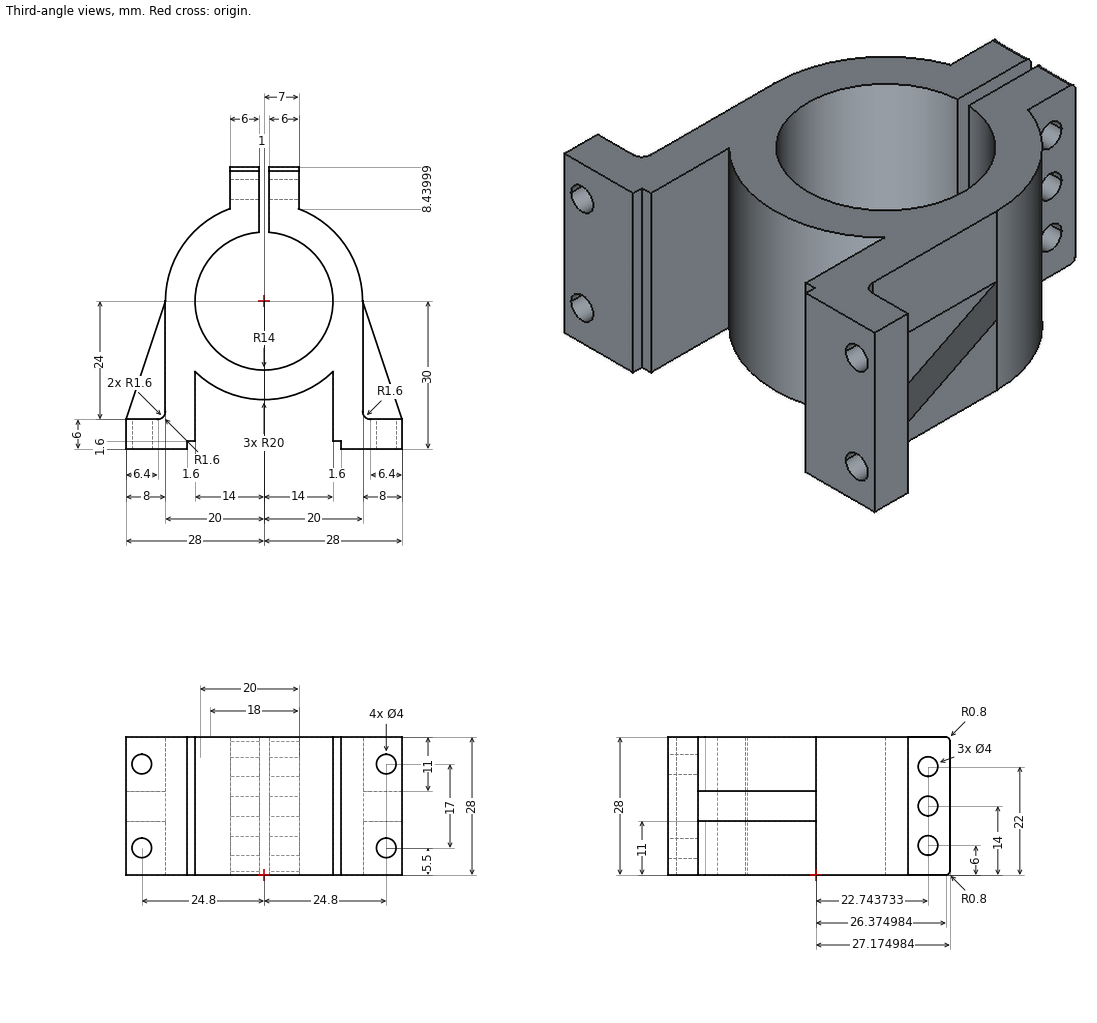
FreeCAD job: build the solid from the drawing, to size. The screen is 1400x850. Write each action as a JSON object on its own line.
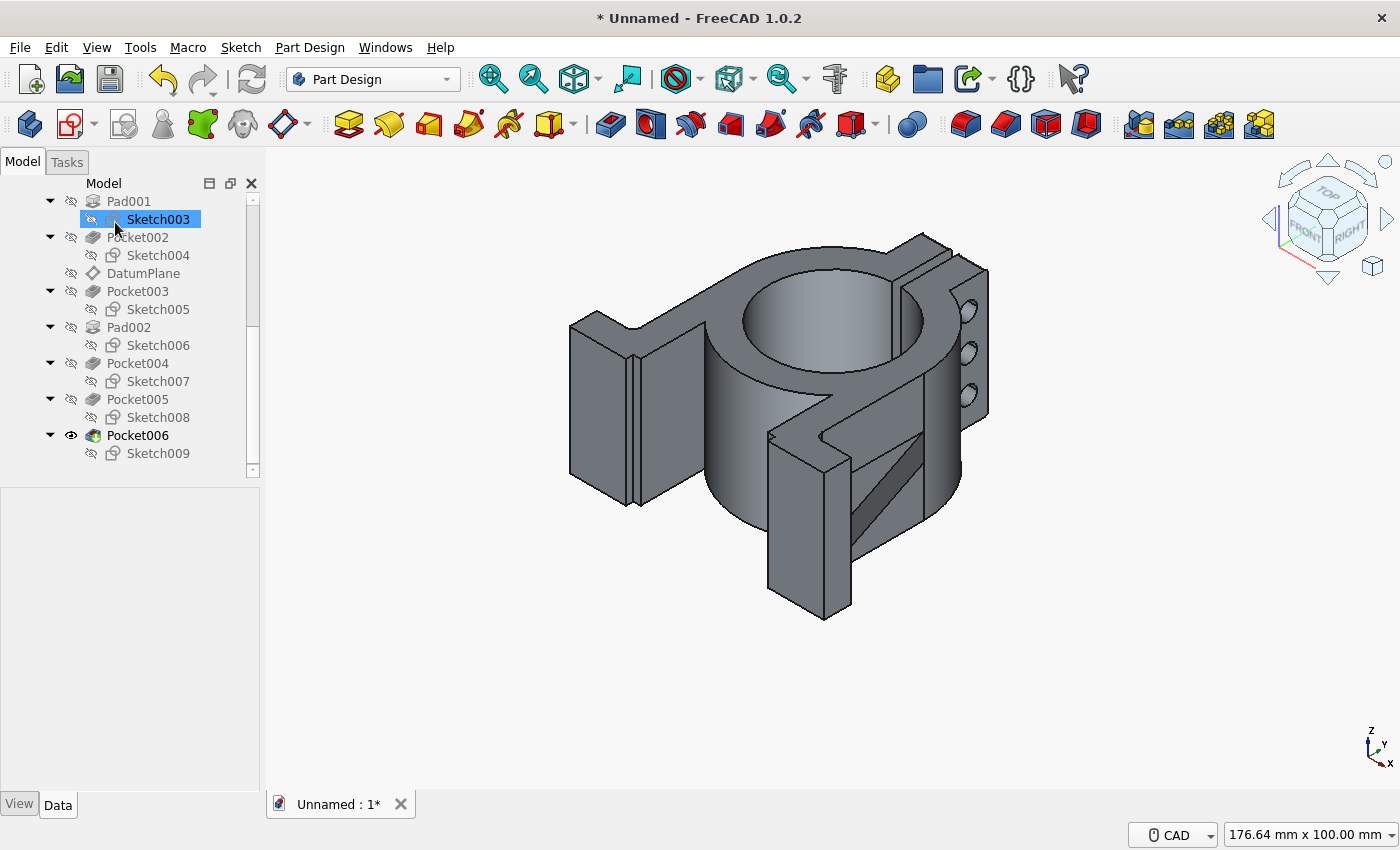
{"action": "key", "text": "4"}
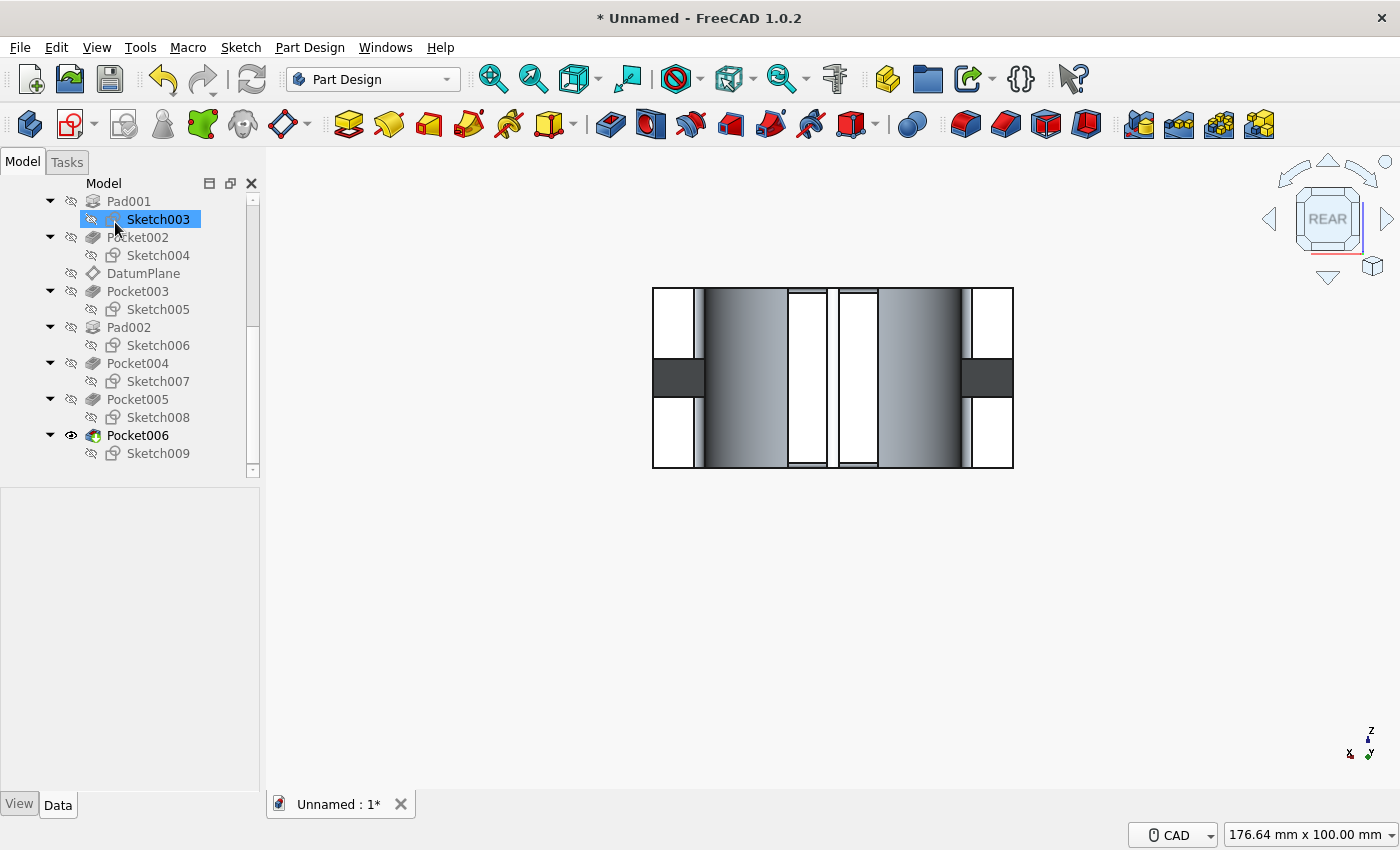
{"action": "left_click", "coordinate": [494, 80]}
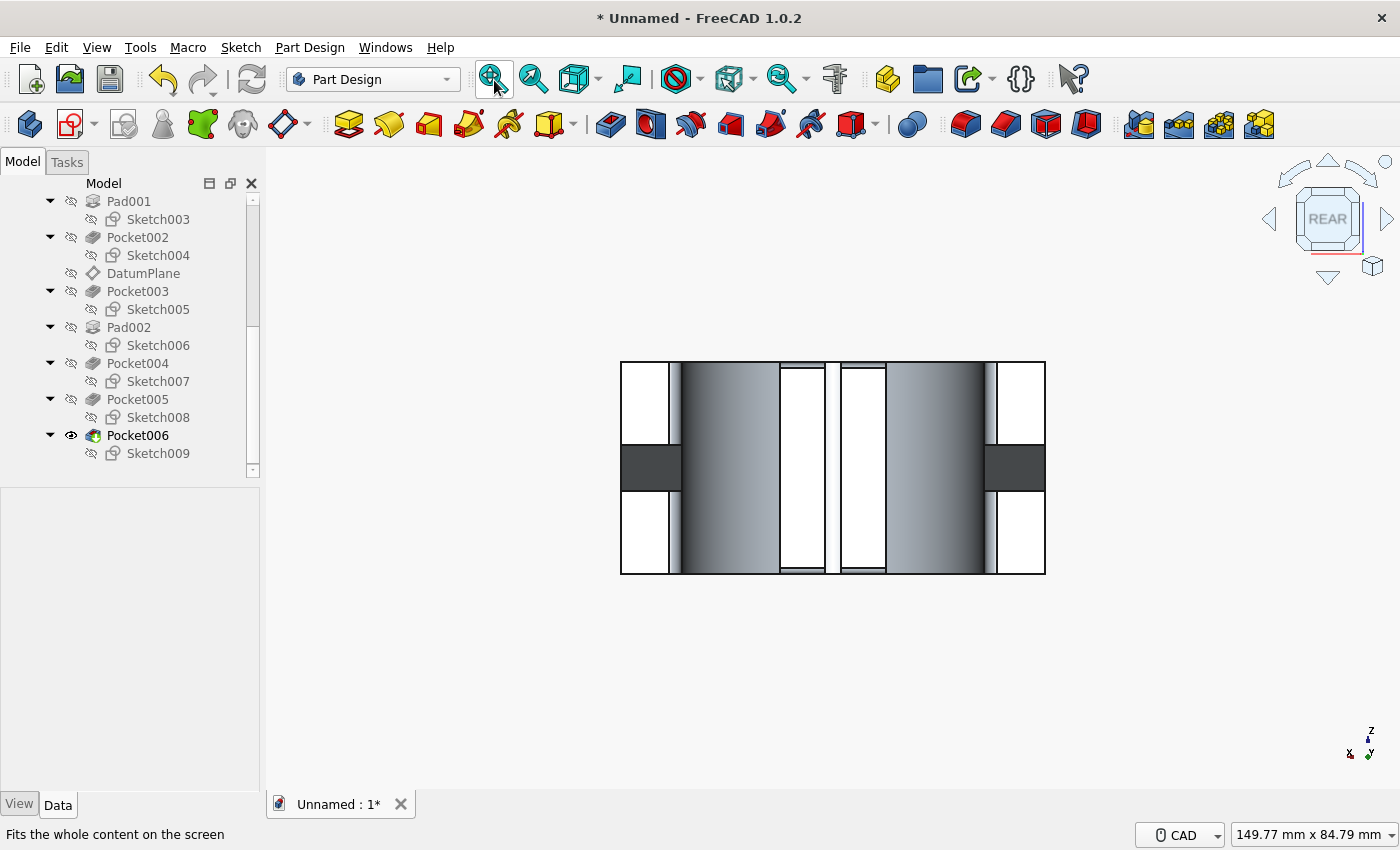
{"action": "left_click", "coordinate": [645, 519]}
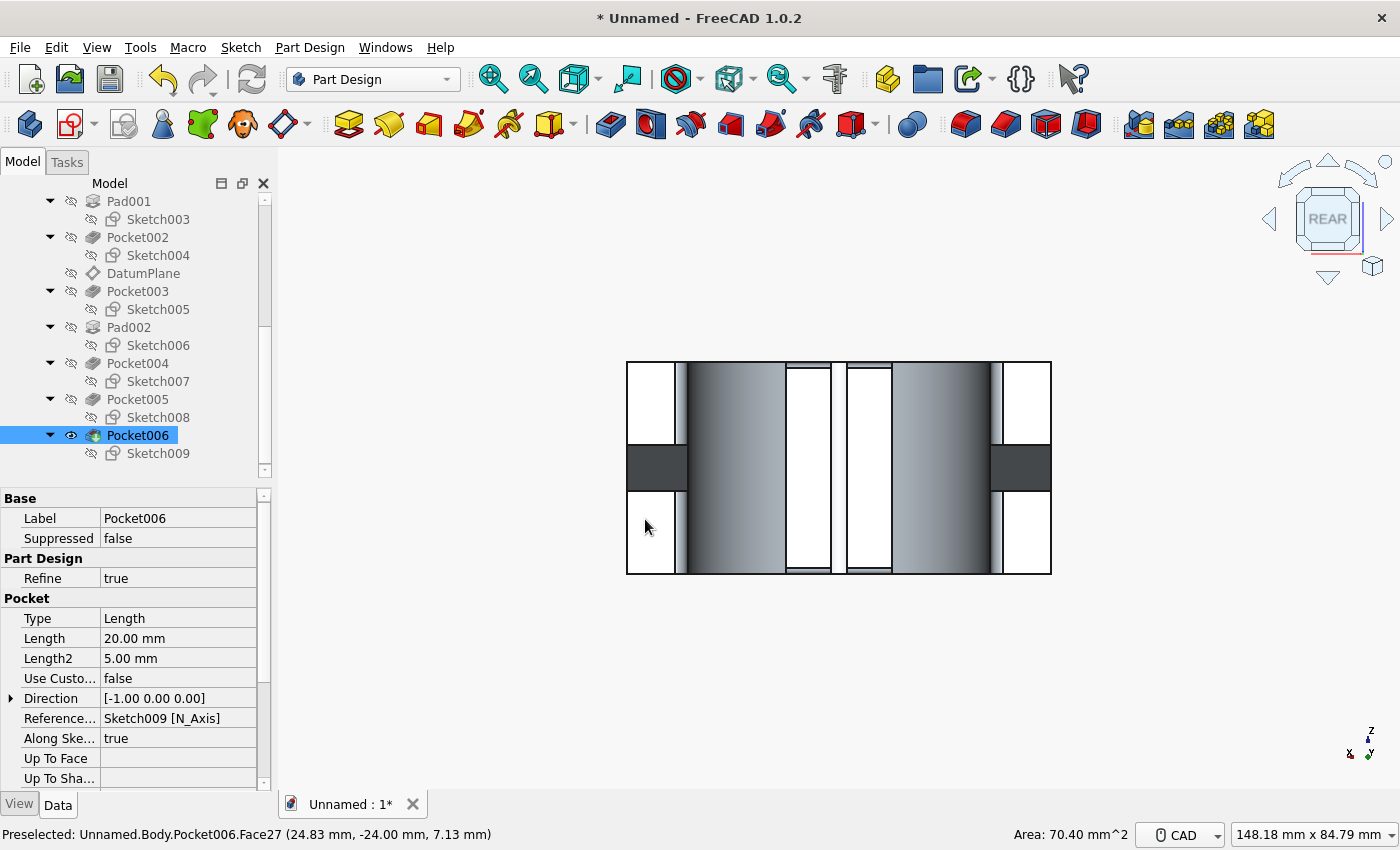
{"action": "left_click", "coordinate": [70, 124]}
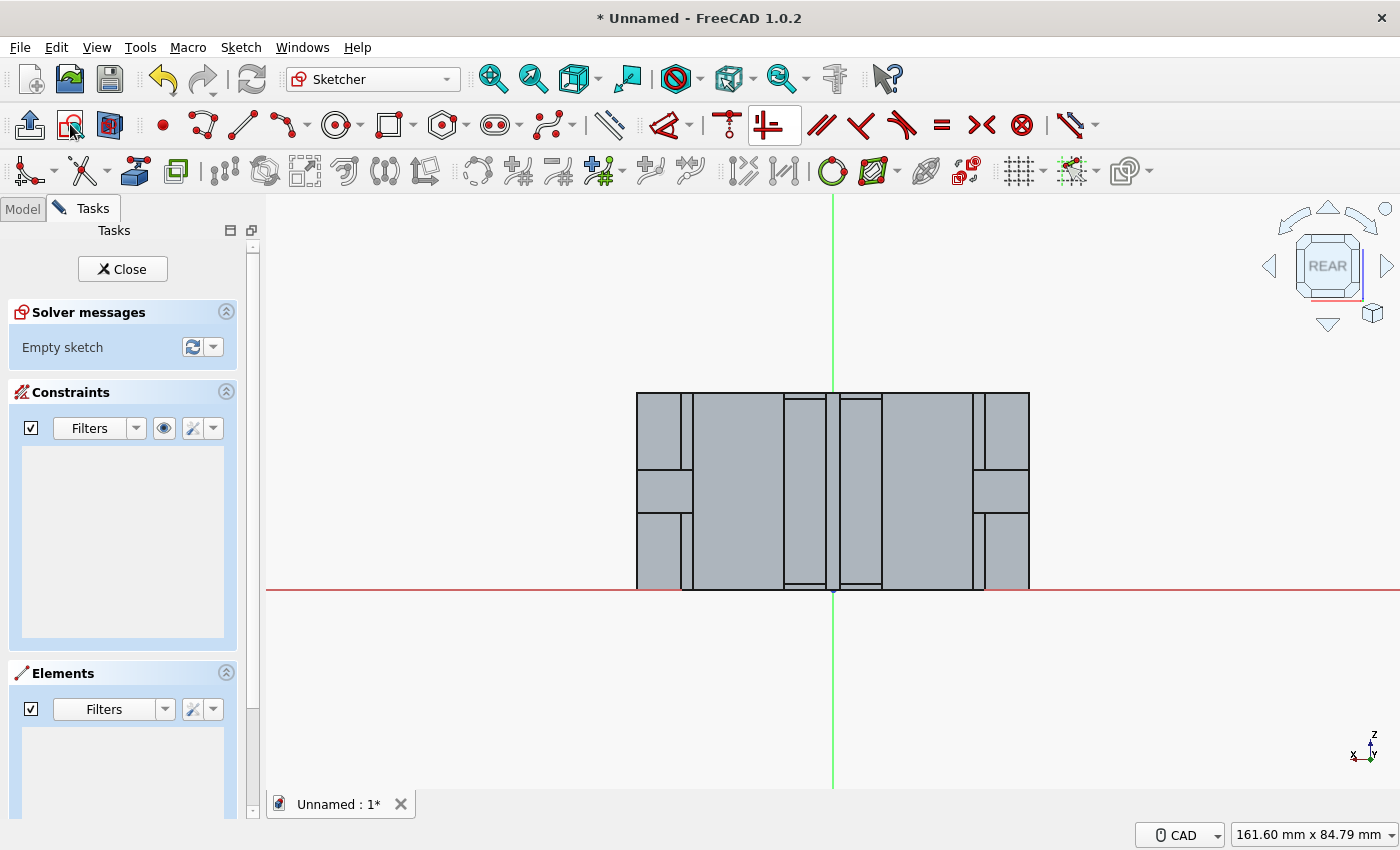
{"action": "scroll", "coordinate": [916, 519], "scroll_direction": "up", "scroll_amount": 3}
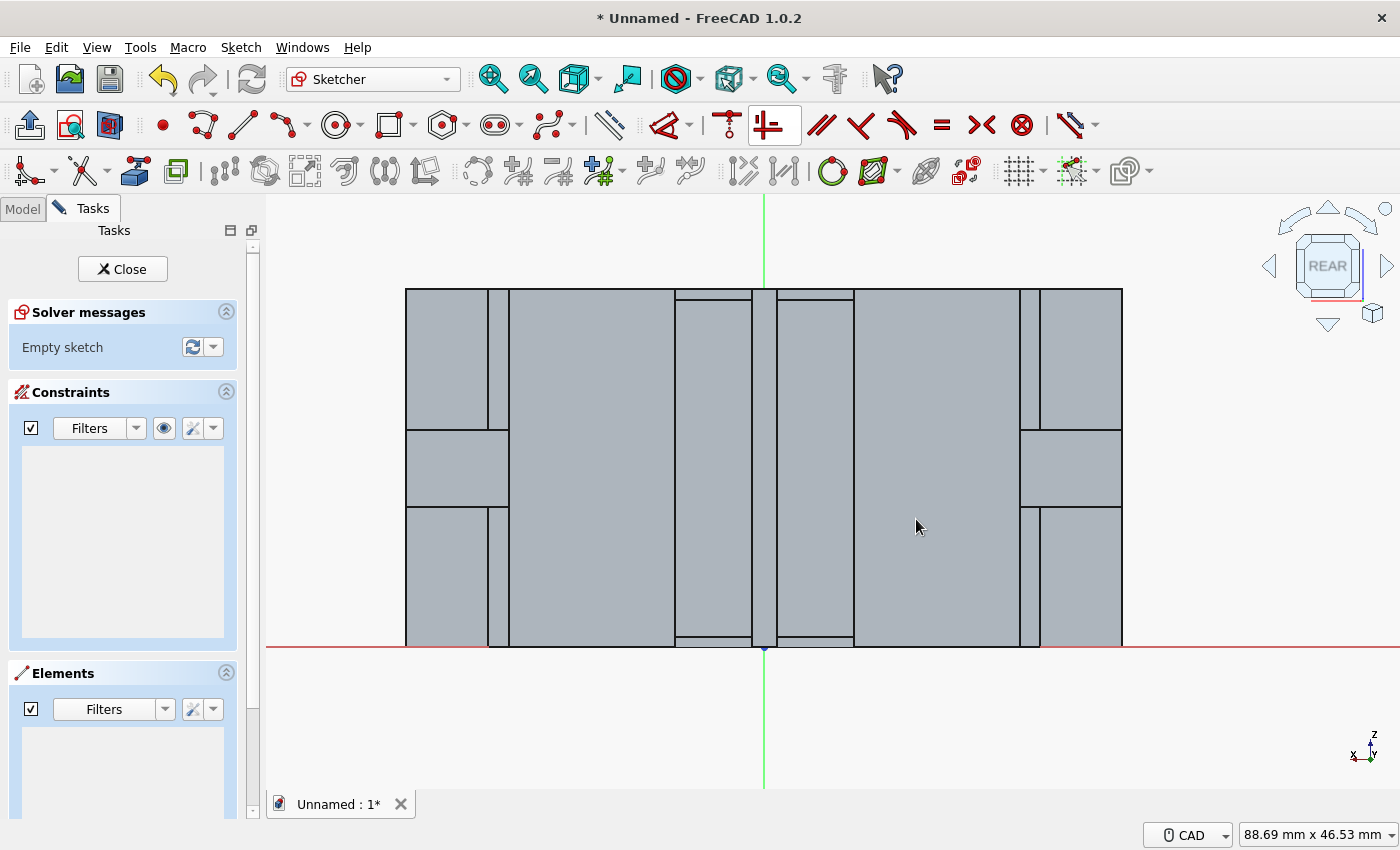
{"action": "left_click", "coordinate": [336, 126]}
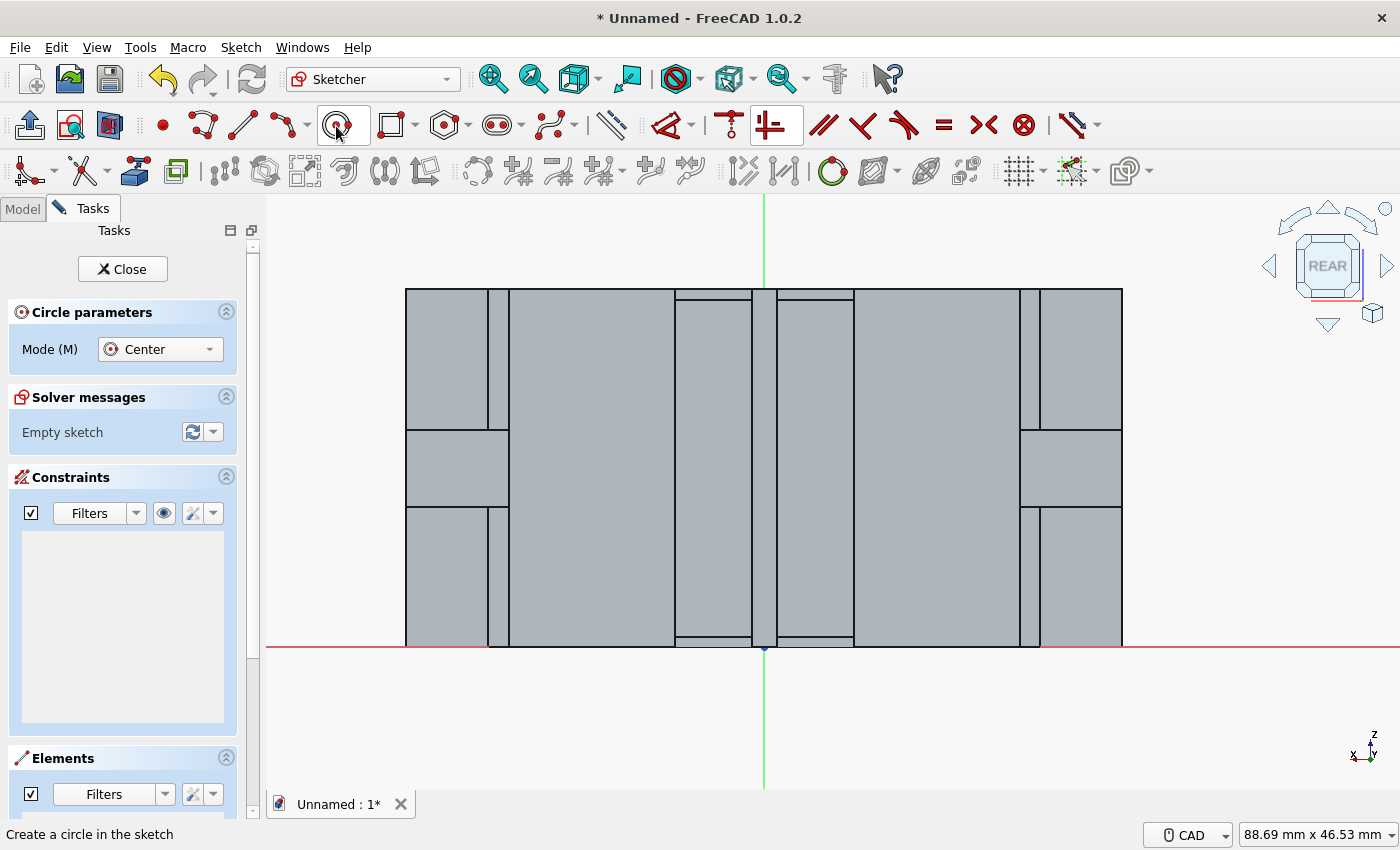
{"action": "left_click", "coordinate": [447, 360]}
{"action": "mouse_move", "coordinate": [465, 342]}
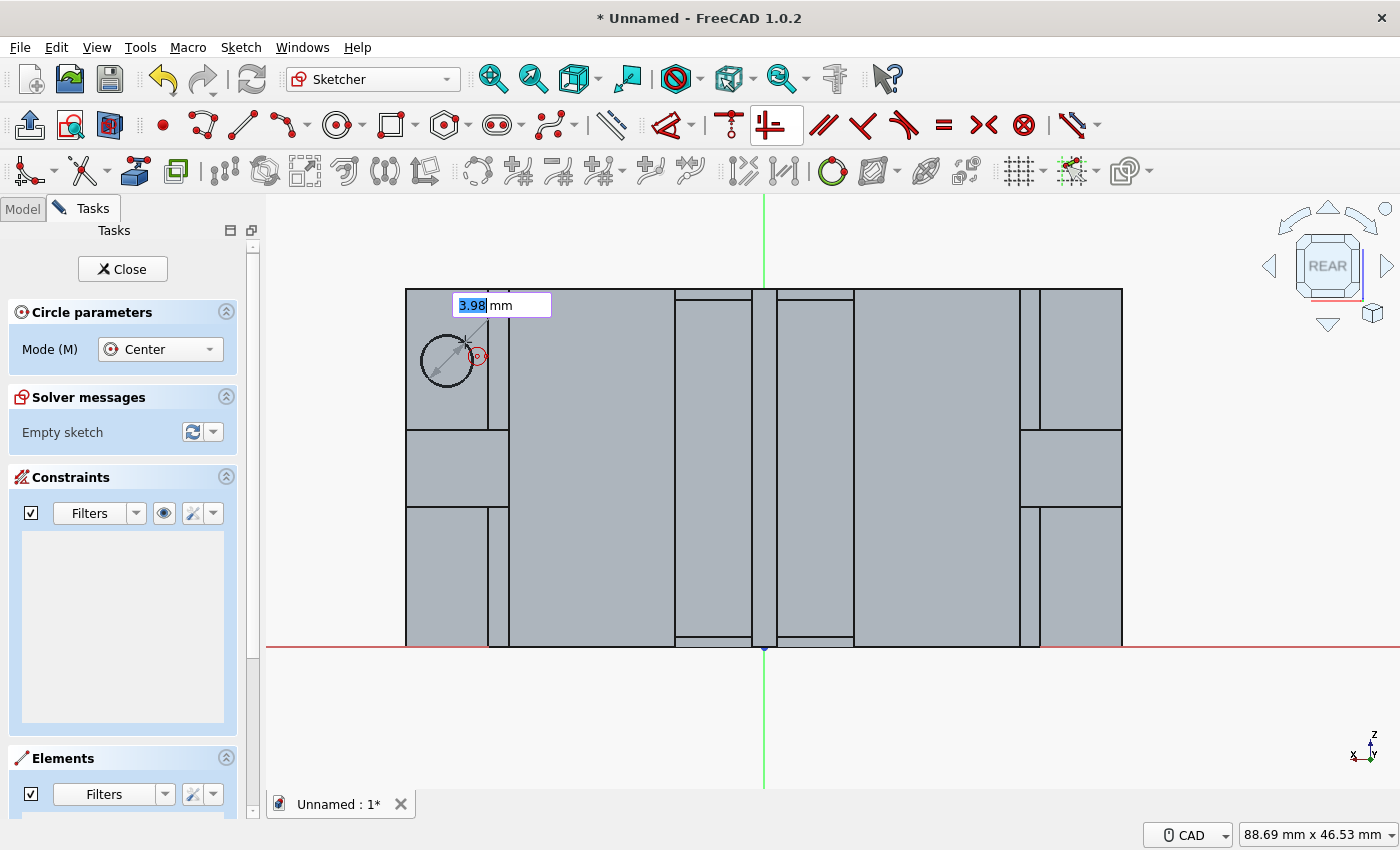
{"action": "type", "text": "4"}
{"action": "key", "text": "Return"}